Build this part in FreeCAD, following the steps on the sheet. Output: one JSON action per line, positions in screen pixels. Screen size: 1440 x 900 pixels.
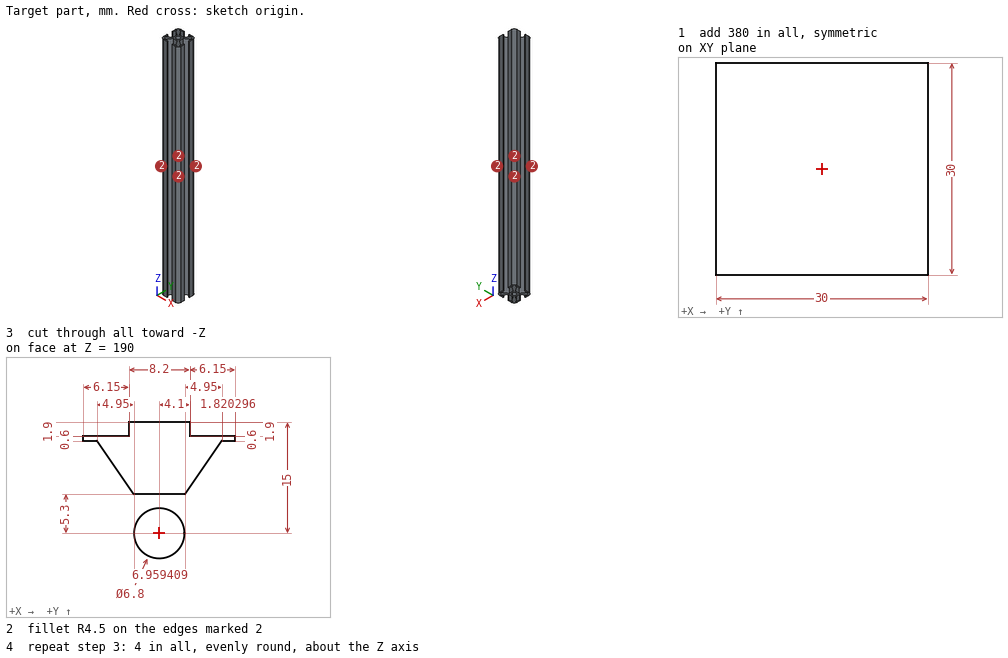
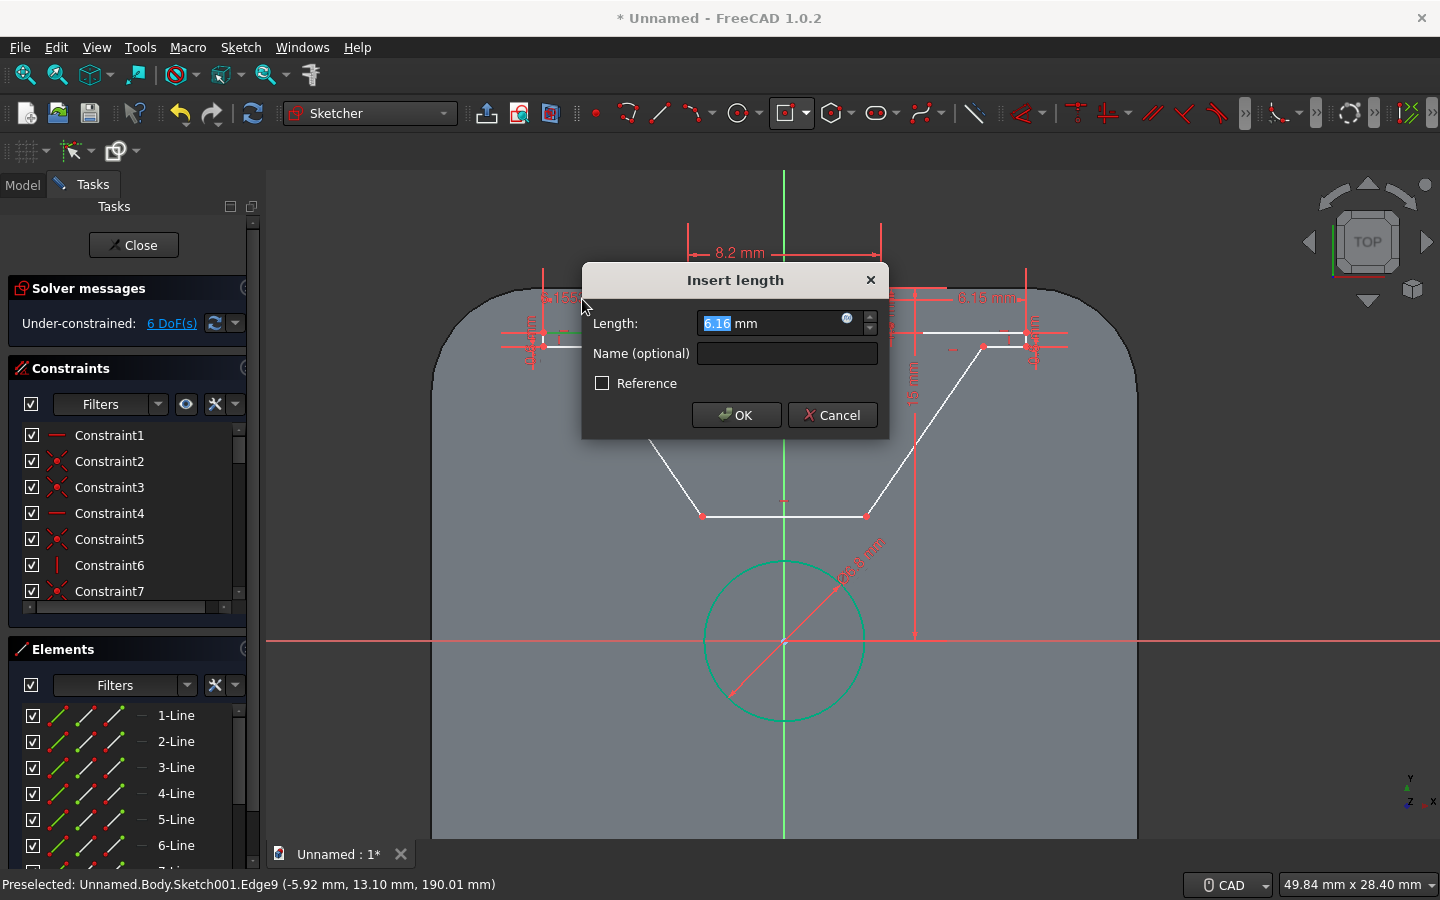
{"action": "type", "text": "6.15"}
{"action": "key", "text": "Return"}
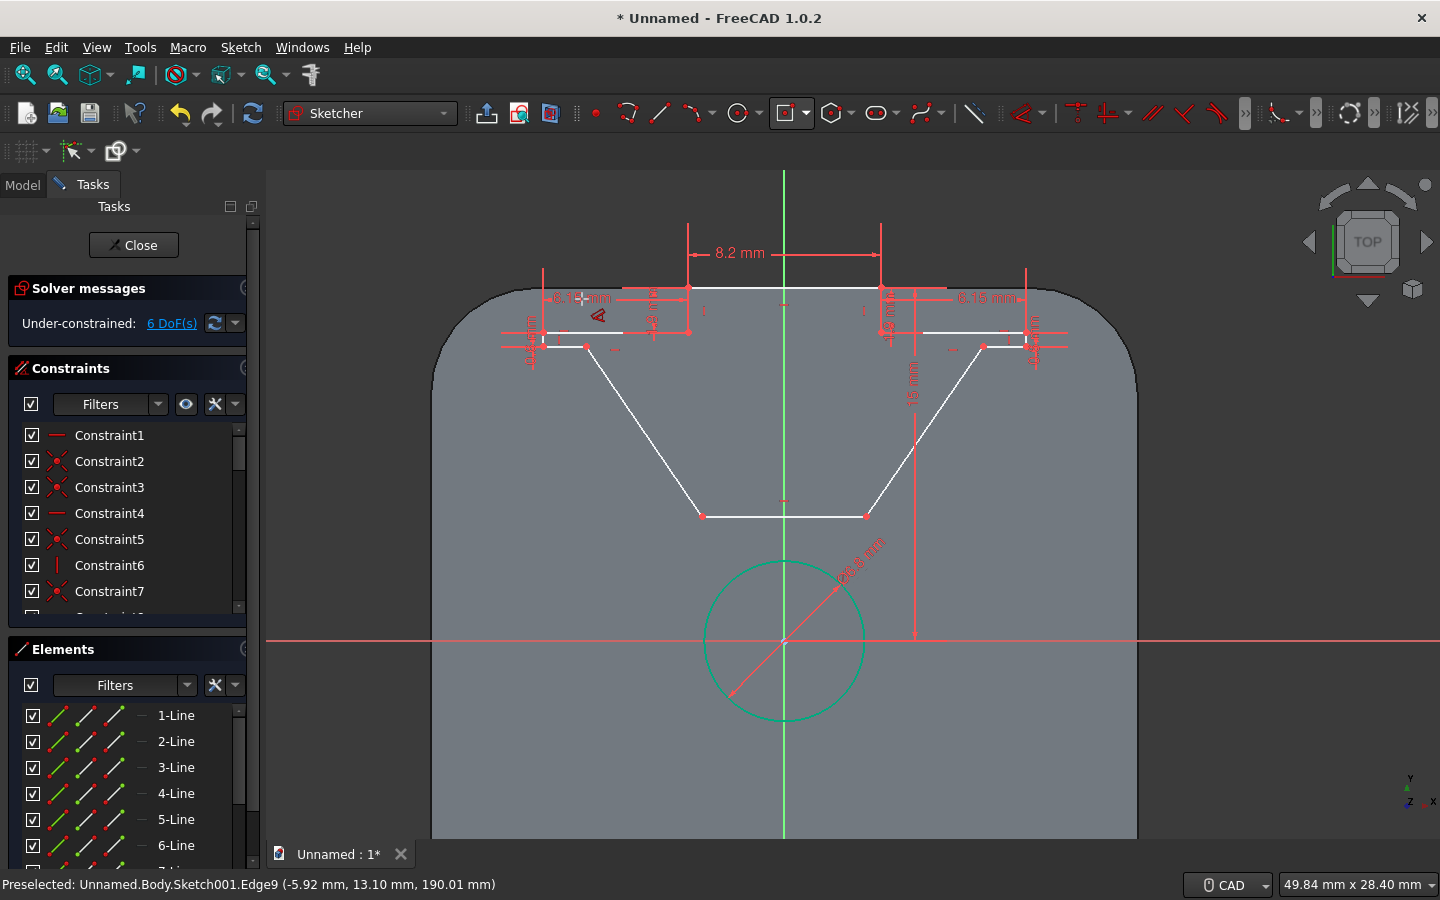
{"action": "left_click", "coordinate": [702, 517]}
{"action": "left_click", "coordinate": [668, 579]}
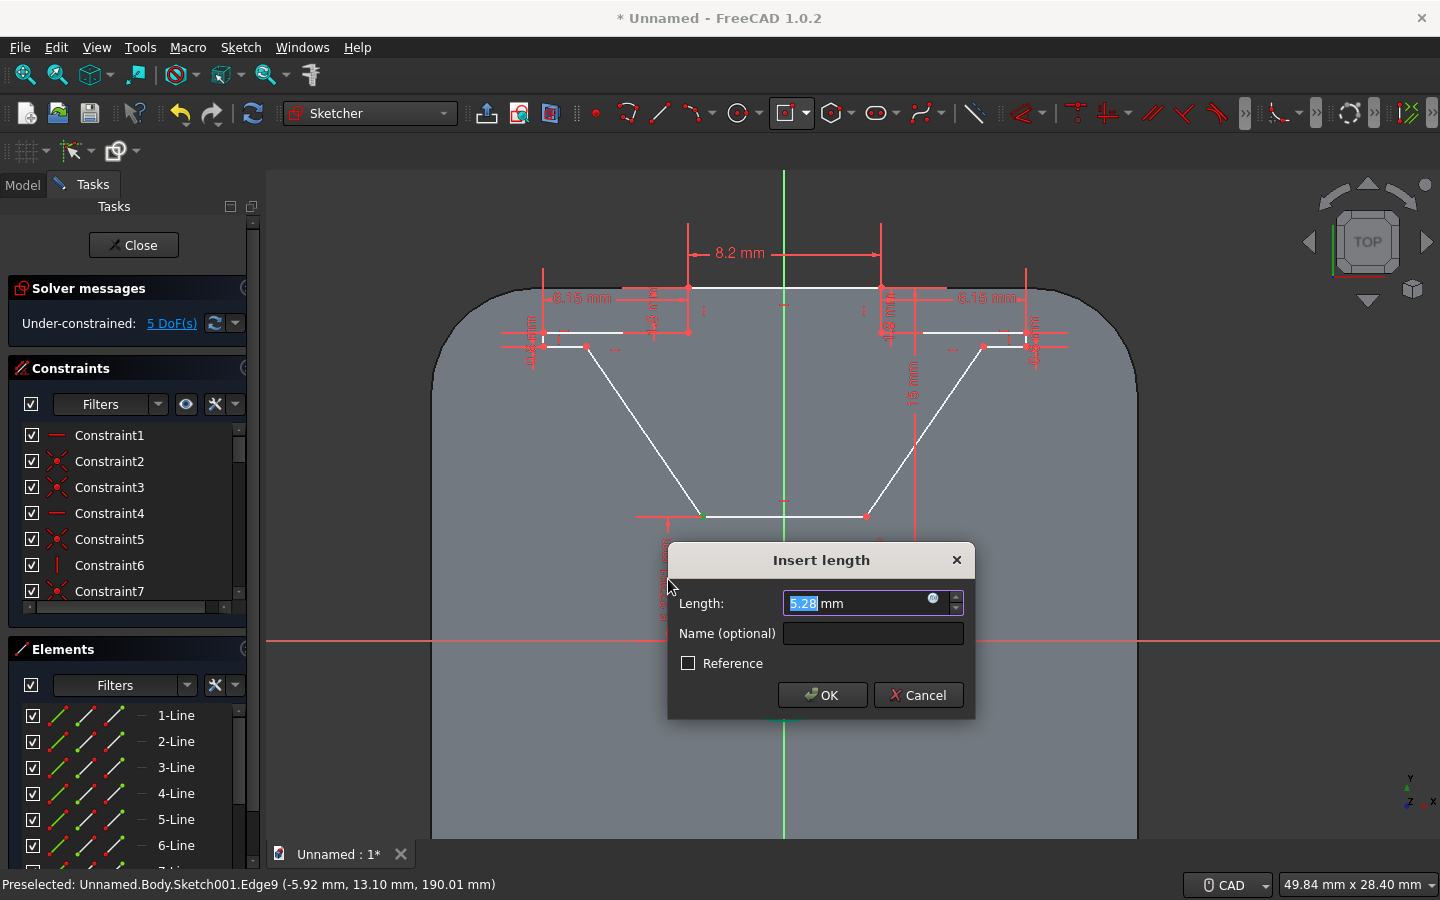
{"action": "type", "text": "5.3"}
{"action": "key", "text": "Return"}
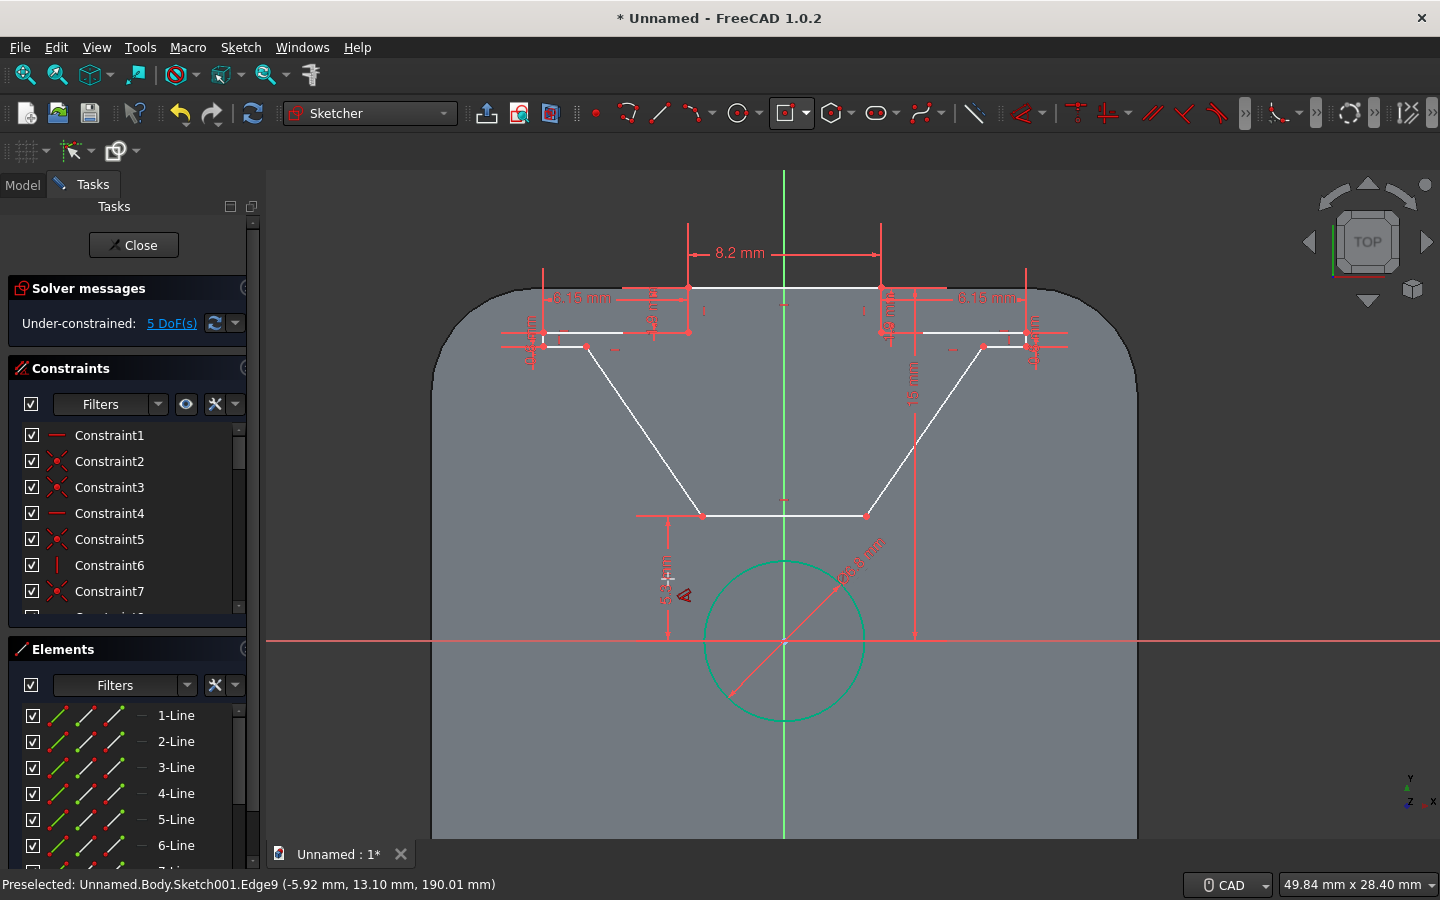
{"action": "left_click", "coordinate": [881, 333]}
{"action": "left_click", "coordinate": [833, 675]}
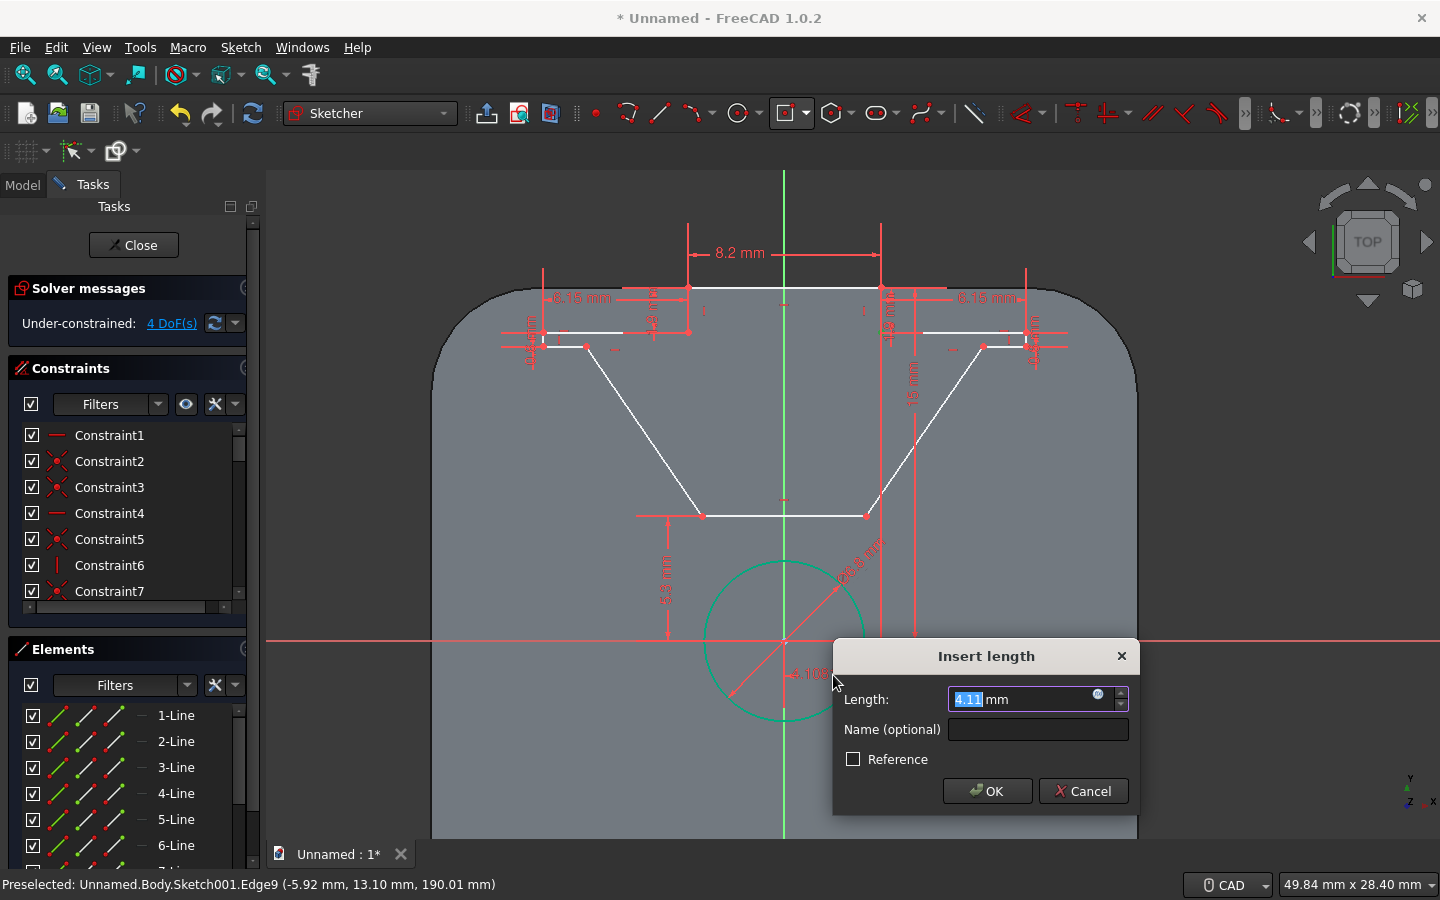
{"action": "type", "text": "4.1"}
{"action": "key", "text": "Return"}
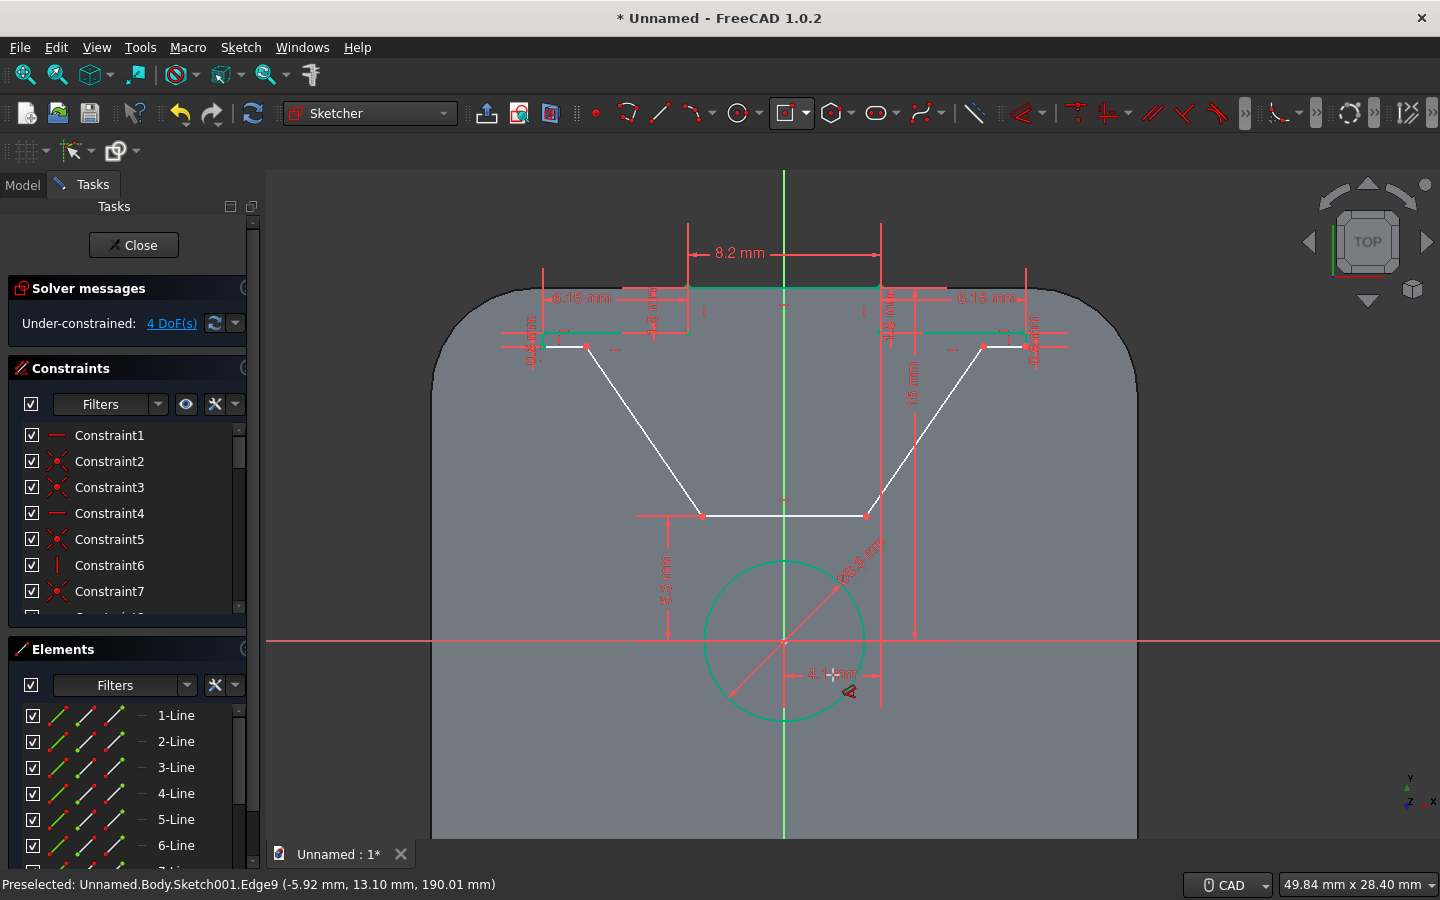
{"action": "left_click", "coordinate": [901, 465]}
{"action": "left_click", "coordinate": [951, 550]}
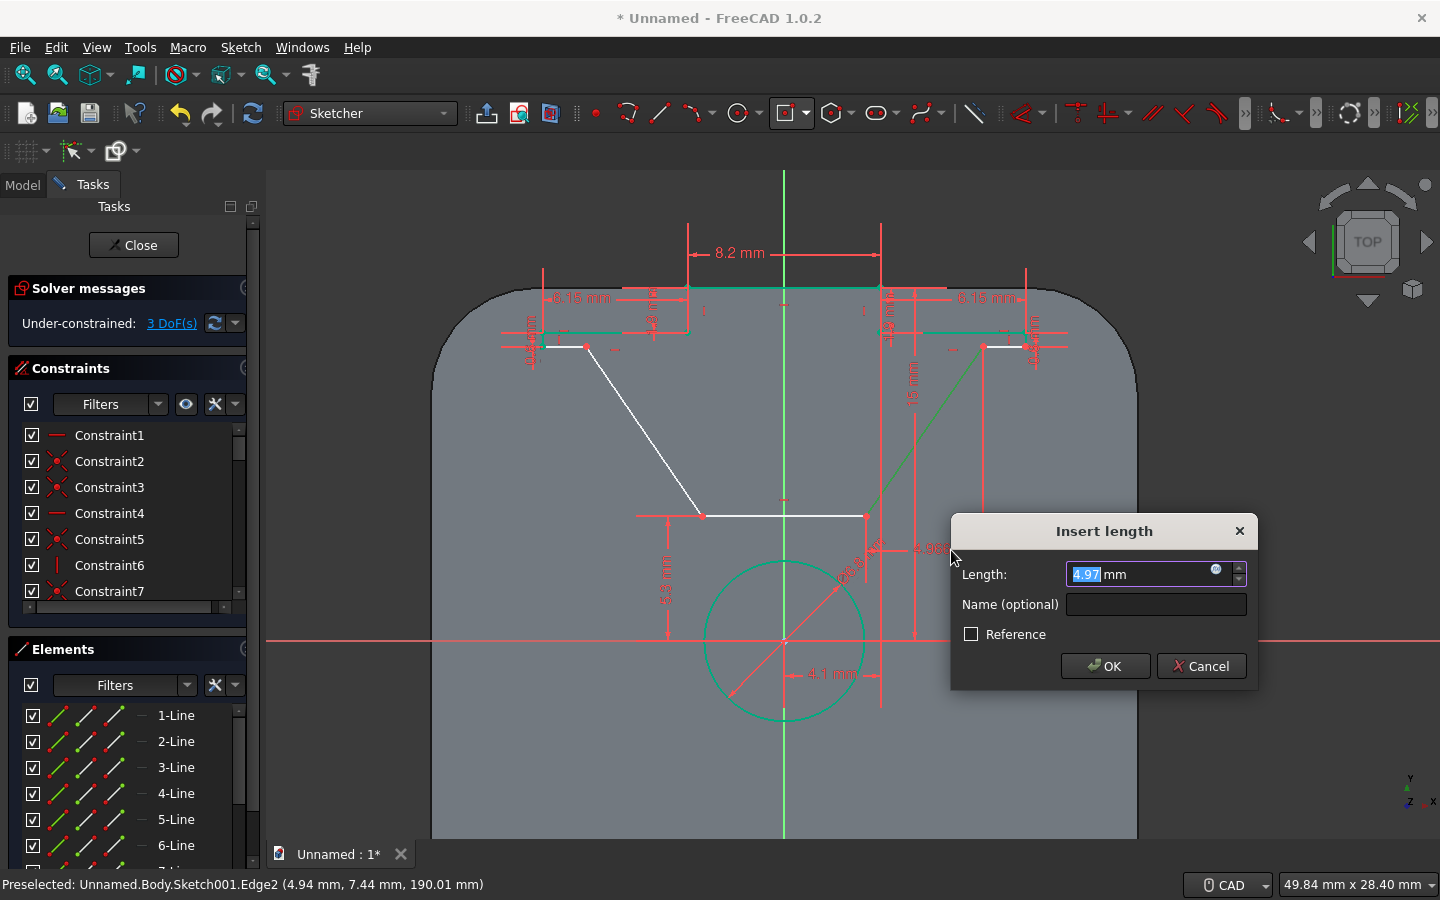
{"action": "type", "text": "4.95"}
{"action": "key", "text": "Return"}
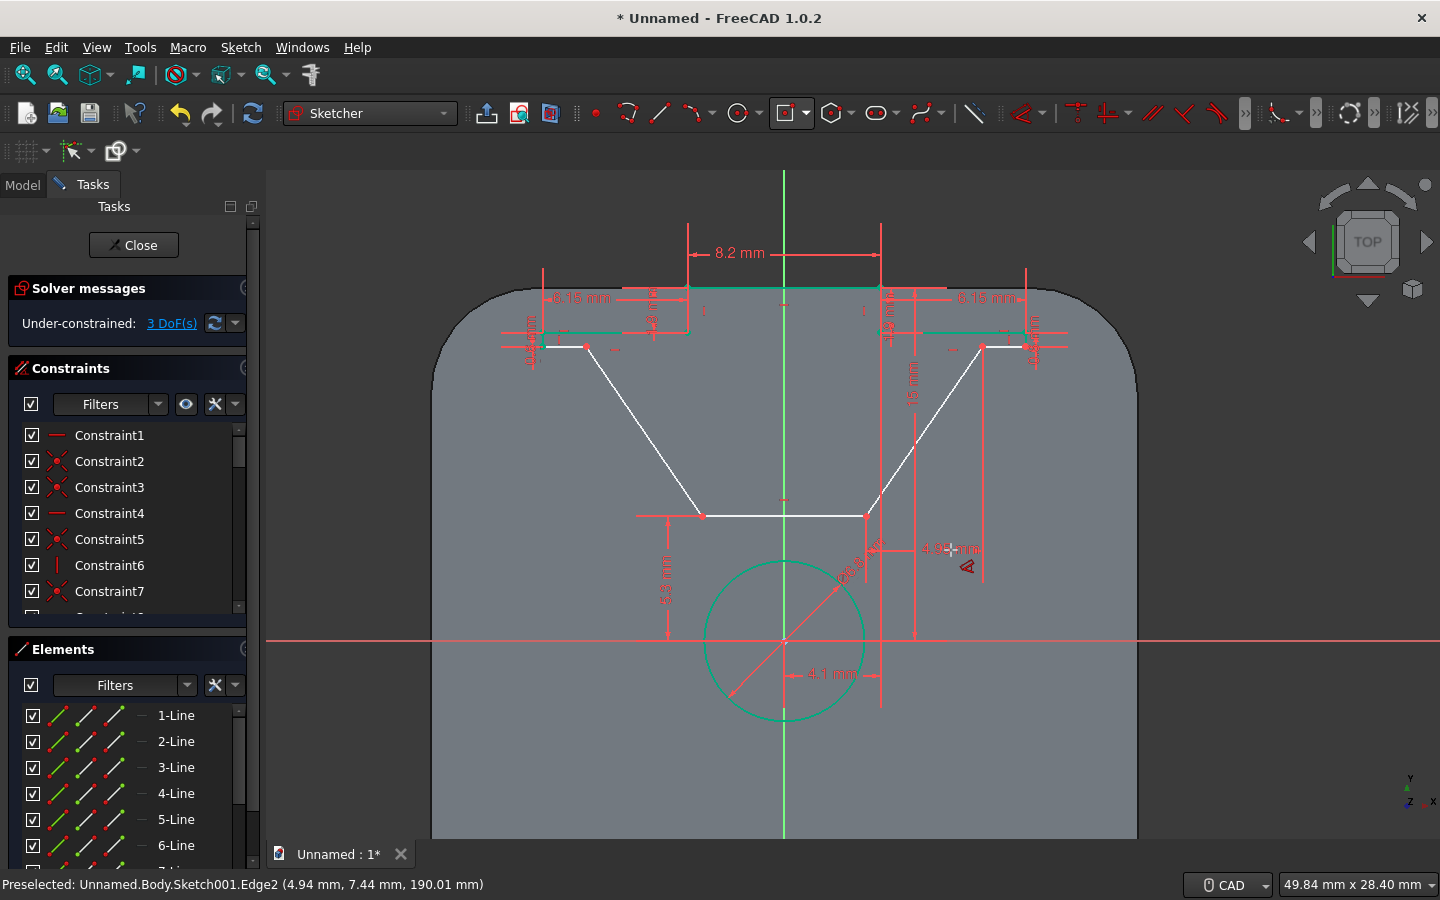
{"action": "left_click", "coordinate": [621, 398]}
{"action": "left_click", "coordinate": [644, 550]}